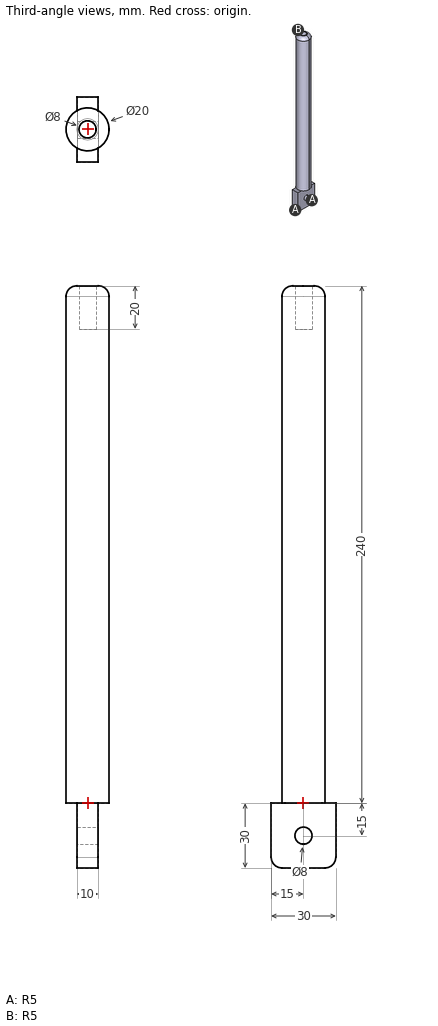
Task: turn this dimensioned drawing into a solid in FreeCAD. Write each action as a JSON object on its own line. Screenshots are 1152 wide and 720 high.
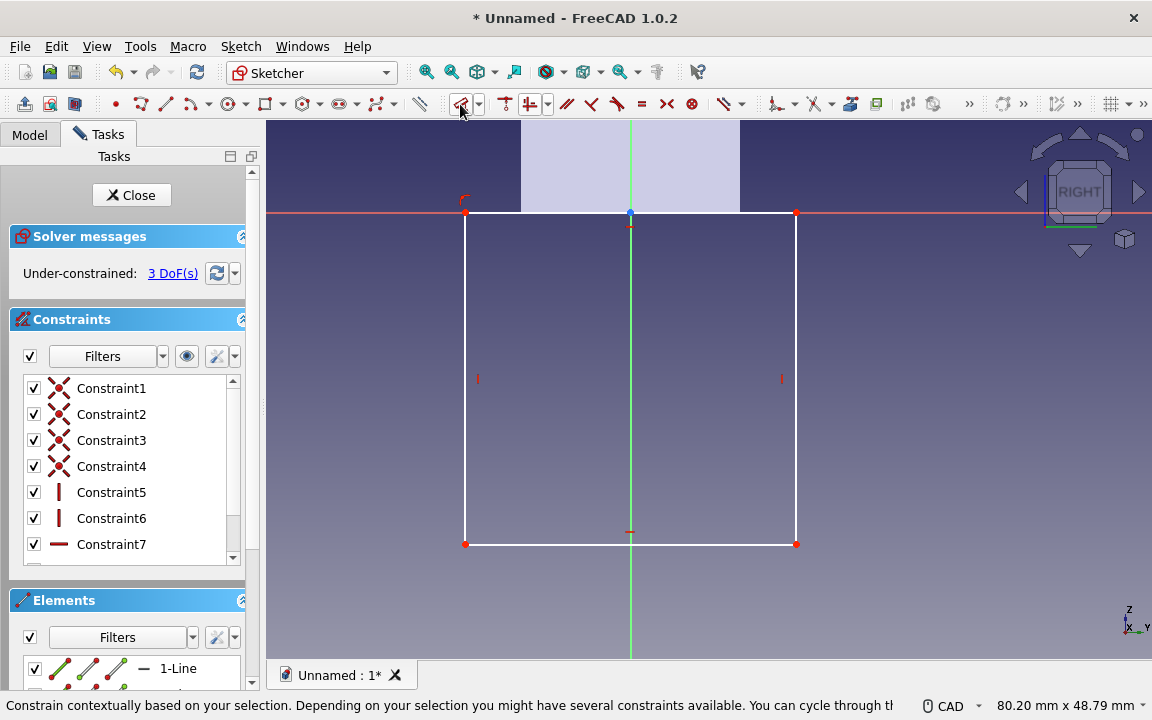
{"action": "left_click", "coordinate": [465, 312]}
{"action": "left_click", "coordinate": [431, 379]}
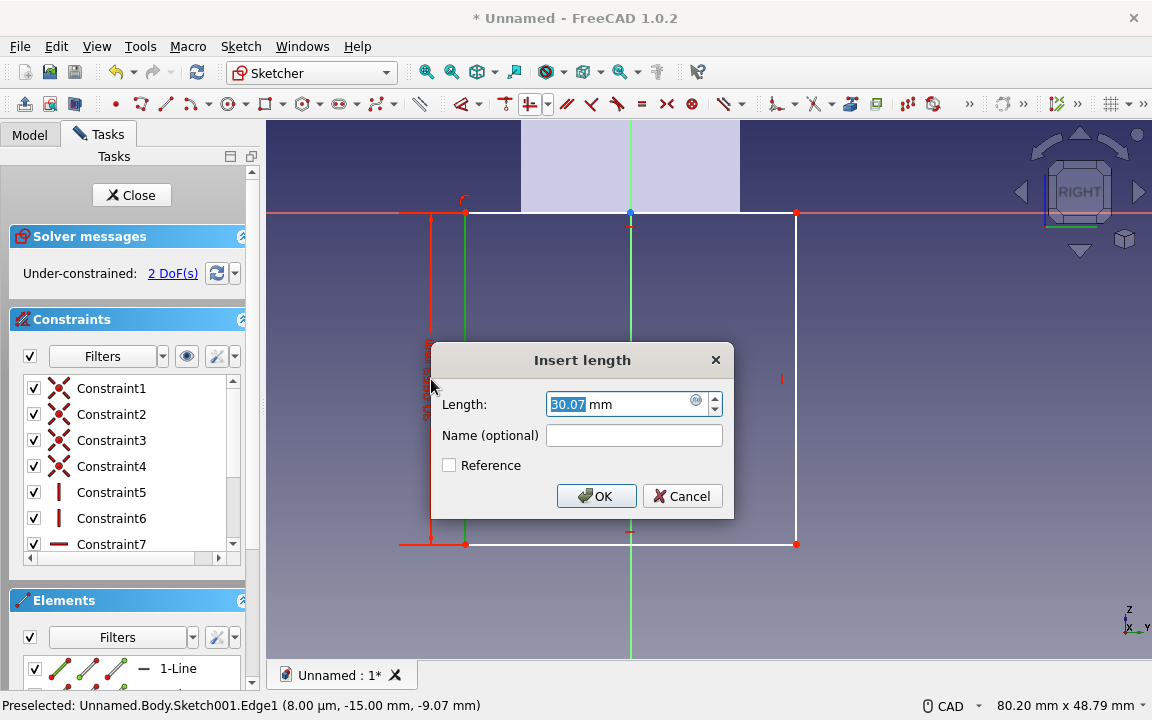
{"action": "type", "text": "30"}
{"action": "key", "text": "Return"}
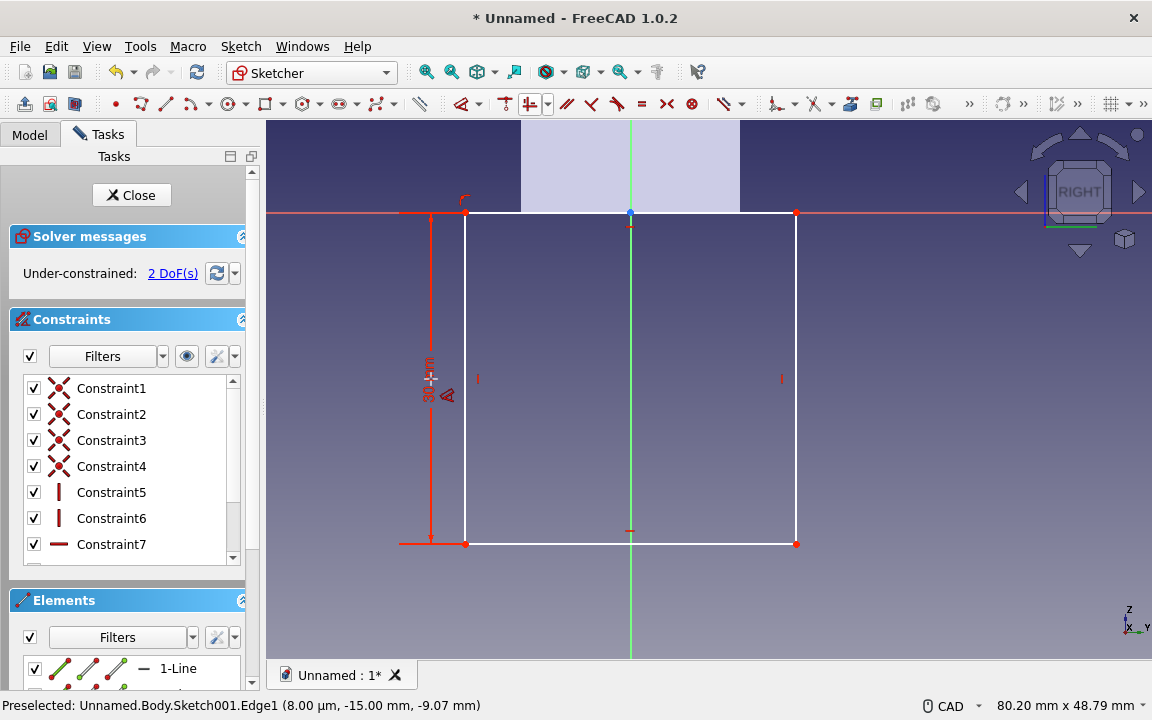
{"action": "left_click", "coordinate": [564, 544]}
{"action": "left_click", "coordinate": [554, 578]}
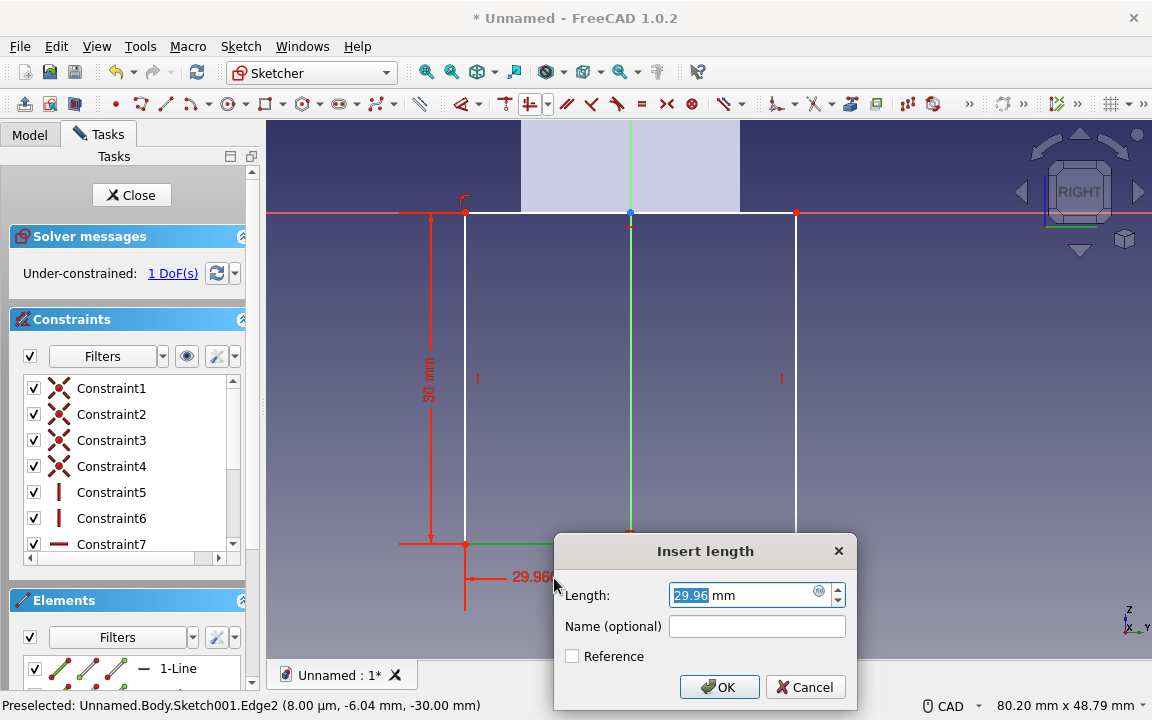
{"action": "type", "text": "30"}
{"action": "key", "text": "Return"}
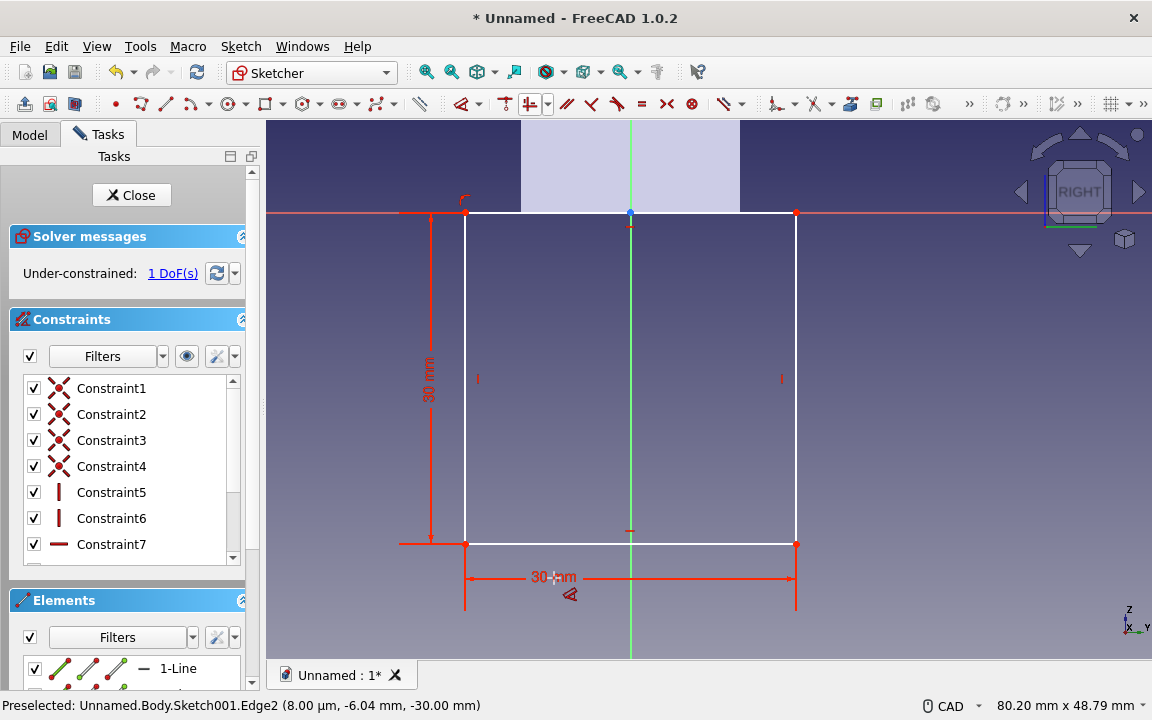
{"action": "left_click", "coordinate": [465, 213]}
{"action": "left_click", "coordinate": [548, 179]}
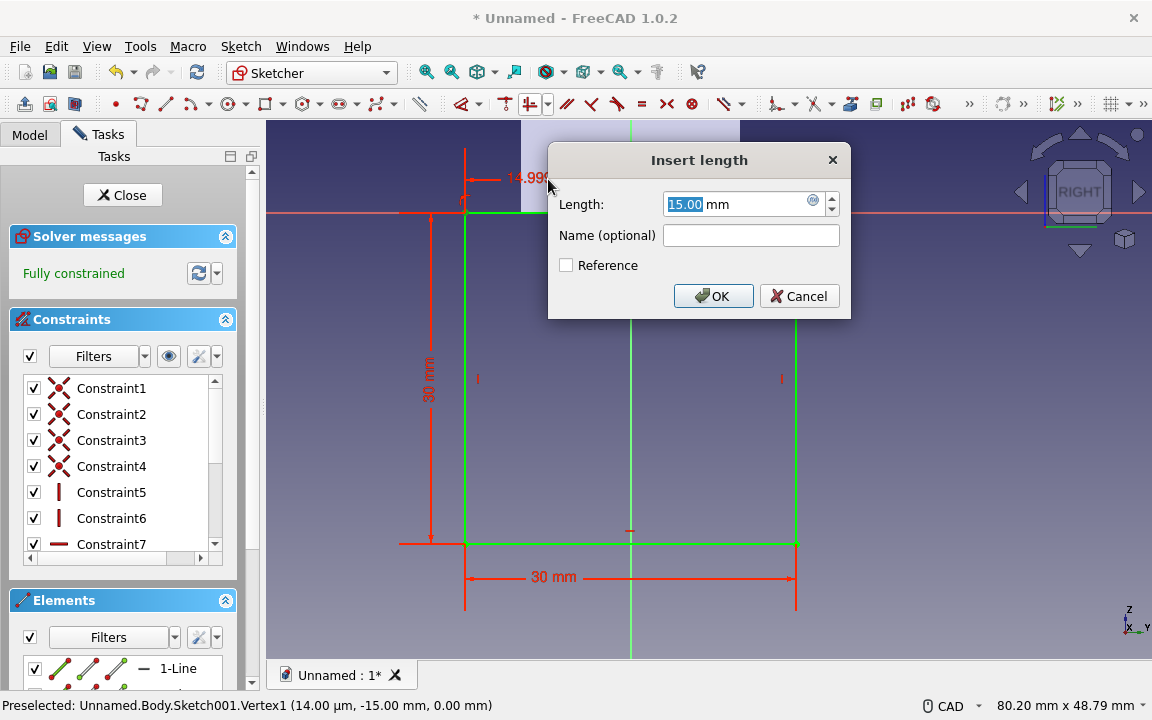
{"action": "type", "text": "15"}
{"action": "key", "text": "Return"}
{"action": "key", "text": "Escape"}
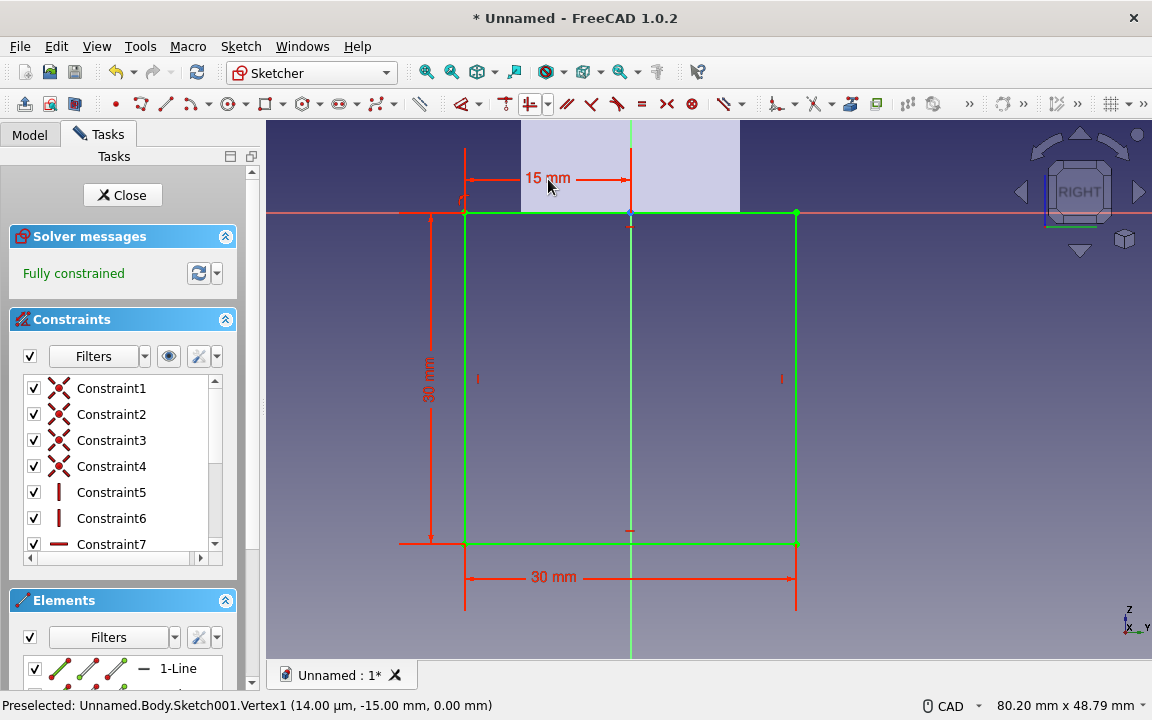
{"action": "left_click", "coordinate": [123, 195]}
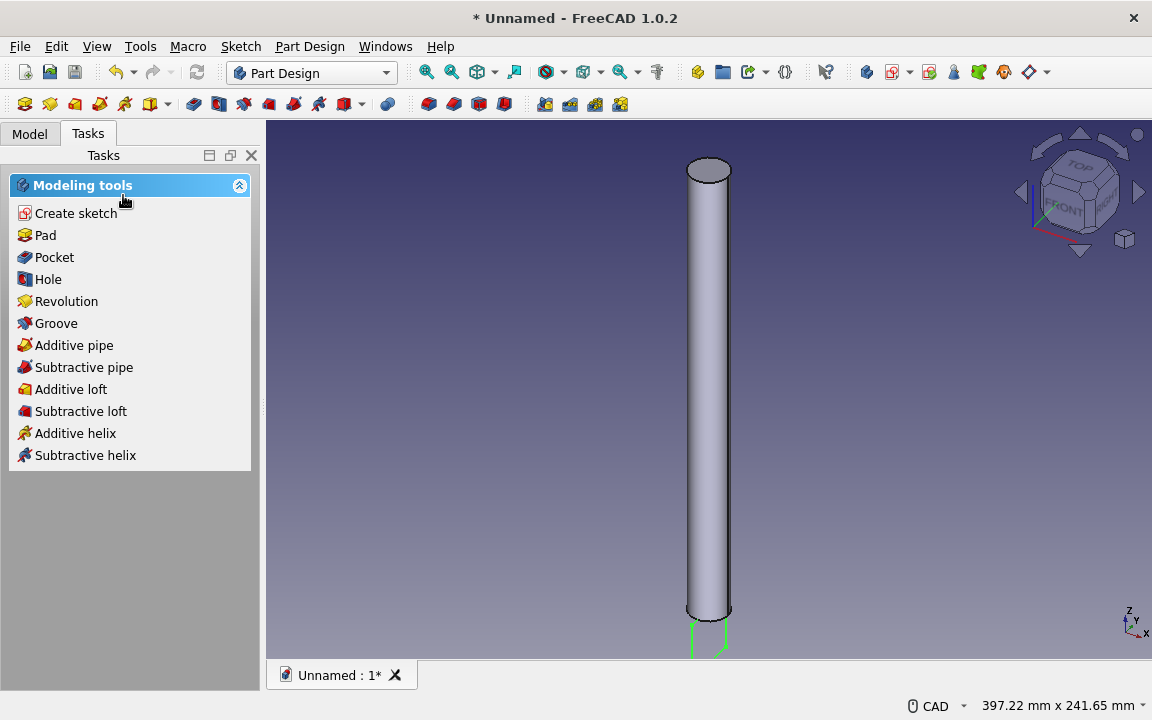
{"action": "left_click", "coordinate": [25, 104]}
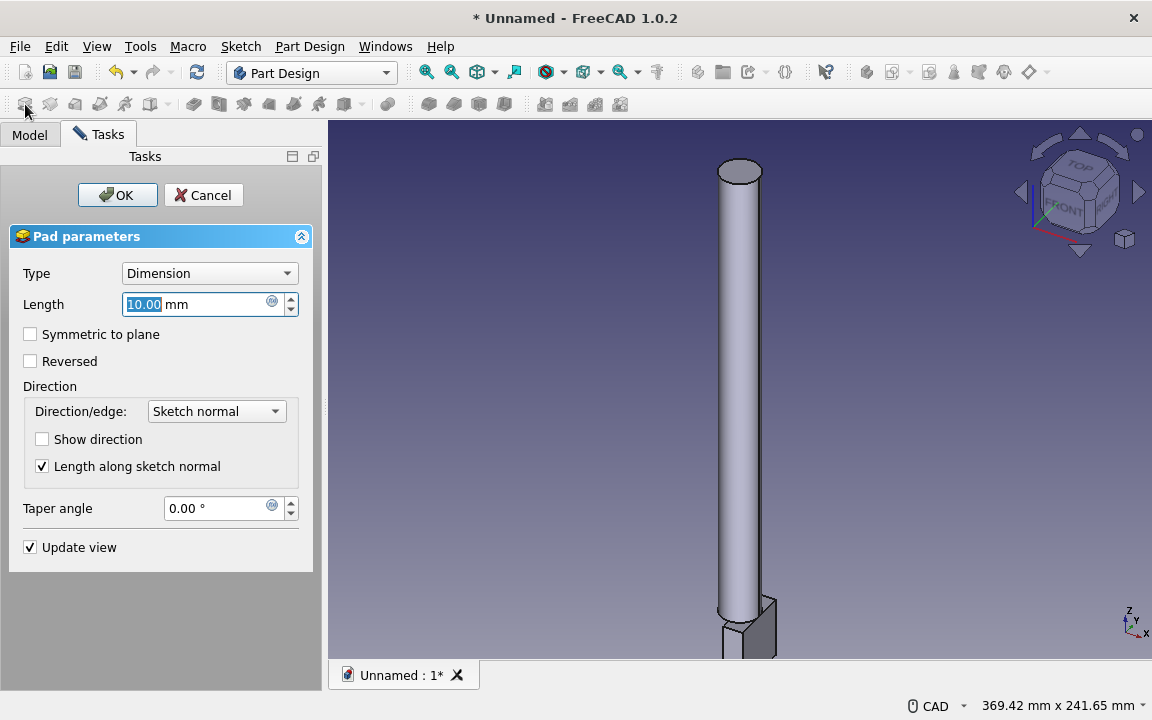
{"action": "type", "text": "10"}
{"action": "key", "text": "Tab"}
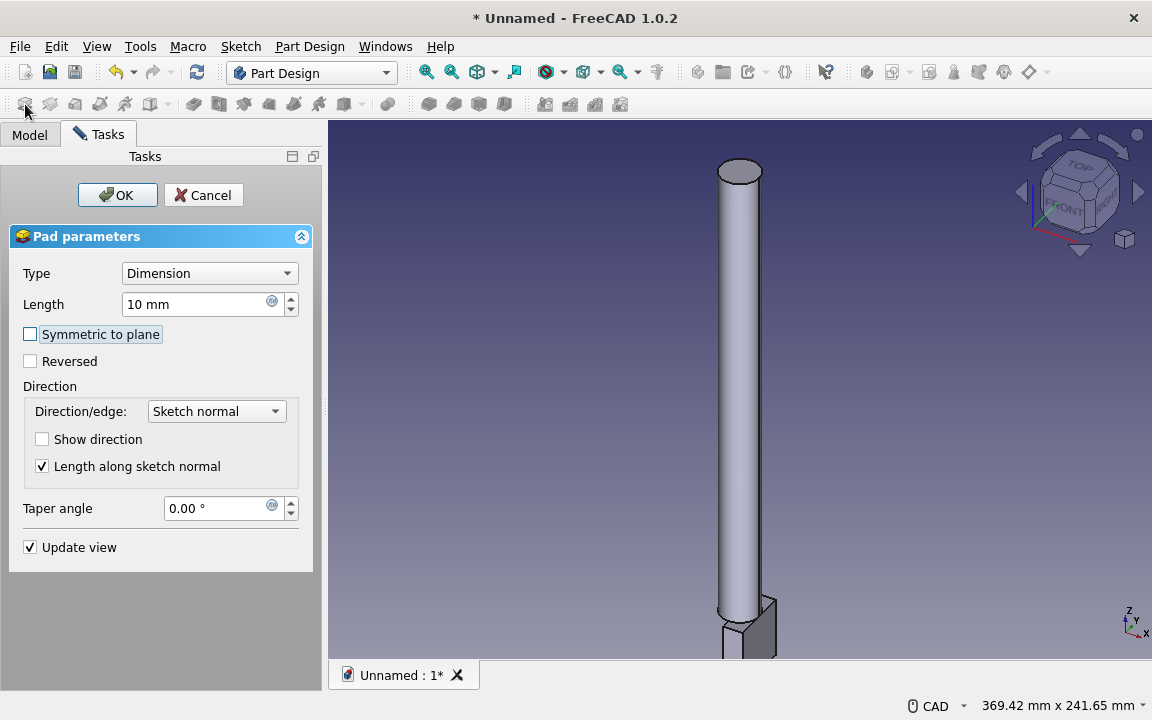
{"action": "left_click", "coordinate": [31, 334]}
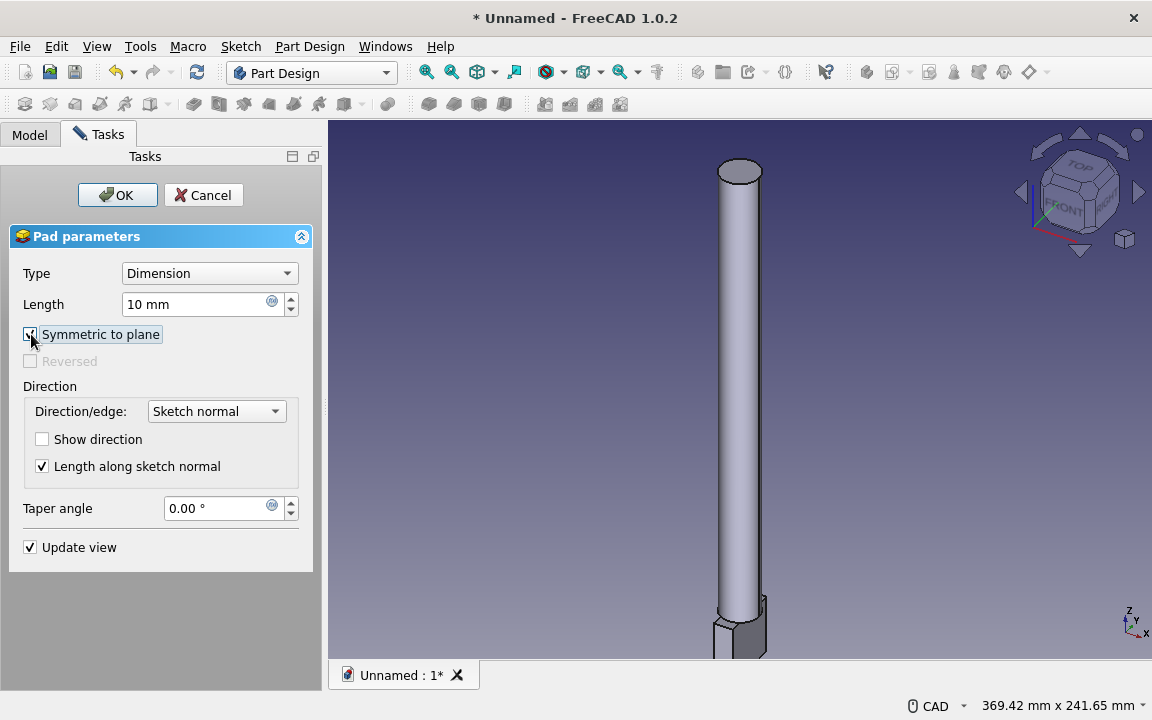
{"action": "left_click", "coordinate": [118, 195]}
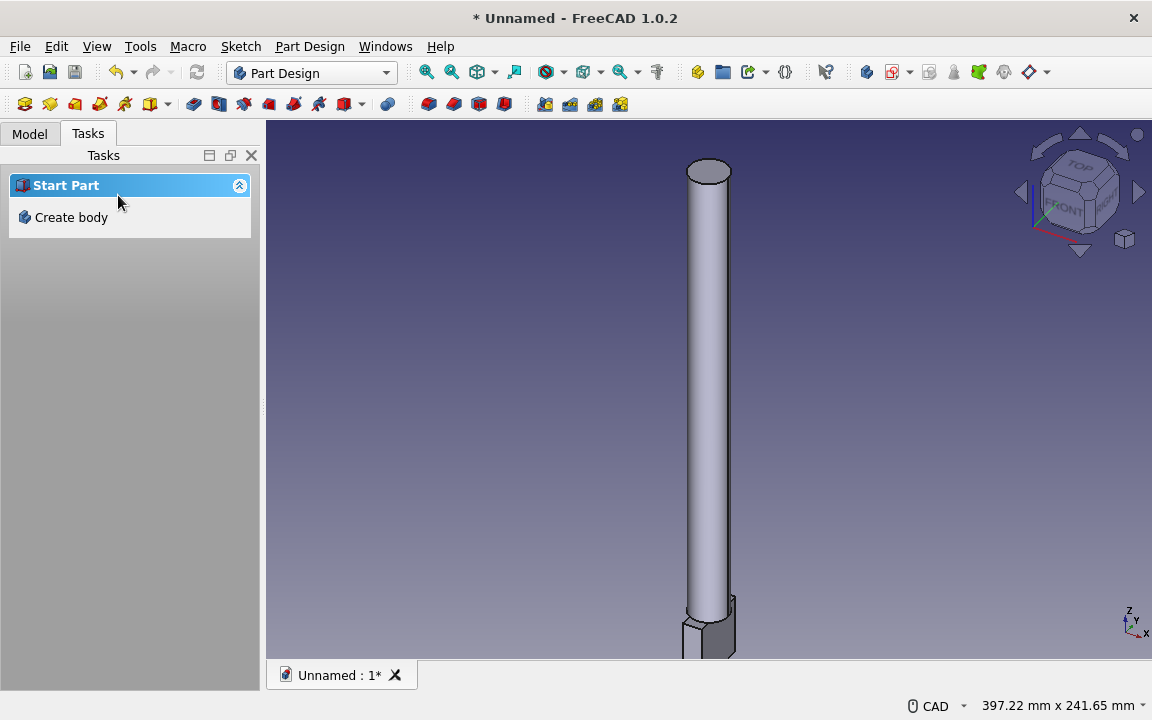
{"action": "key", "text": "v f"}